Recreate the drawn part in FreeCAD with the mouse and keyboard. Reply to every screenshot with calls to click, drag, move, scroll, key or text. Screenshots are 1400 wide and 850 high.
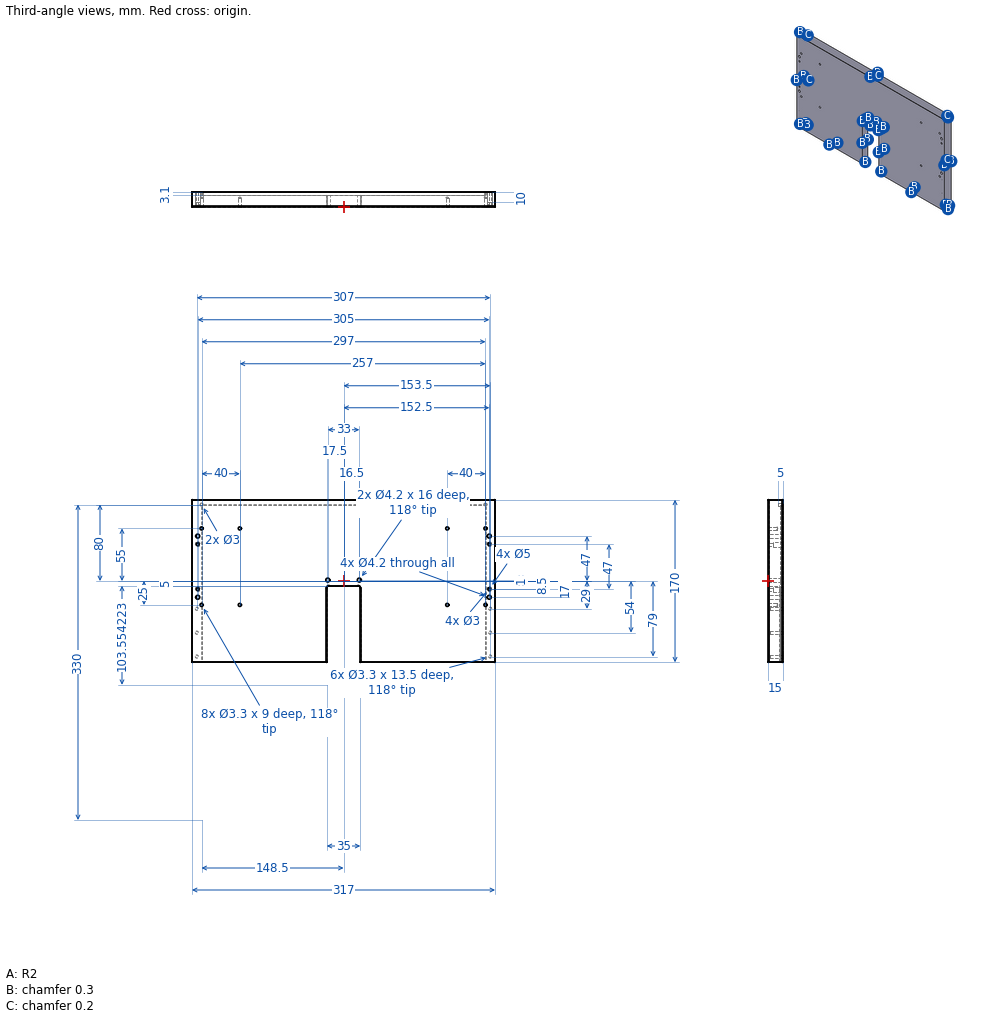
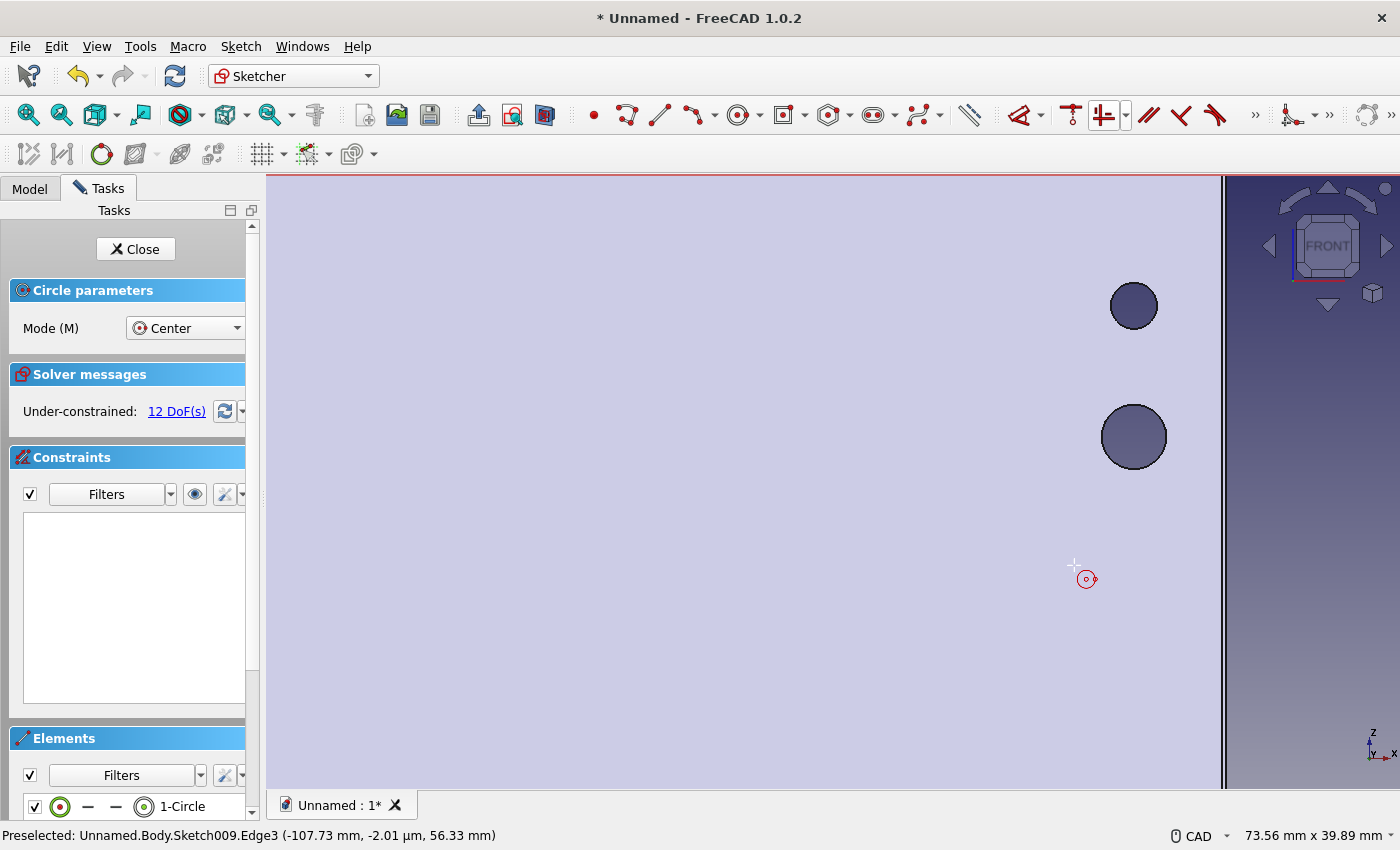
scroll(1075, 566, down, 10)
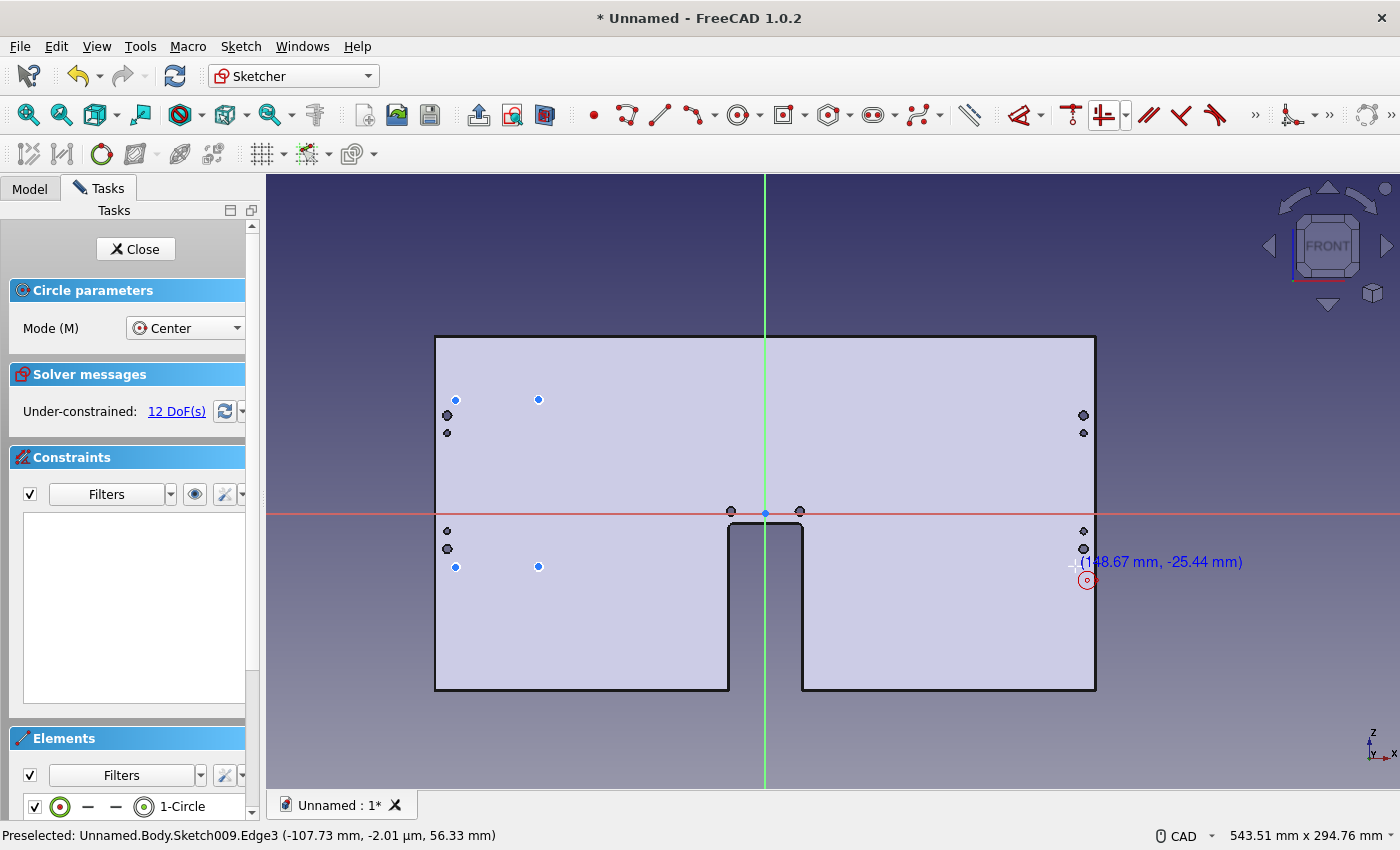
click(1075, 566)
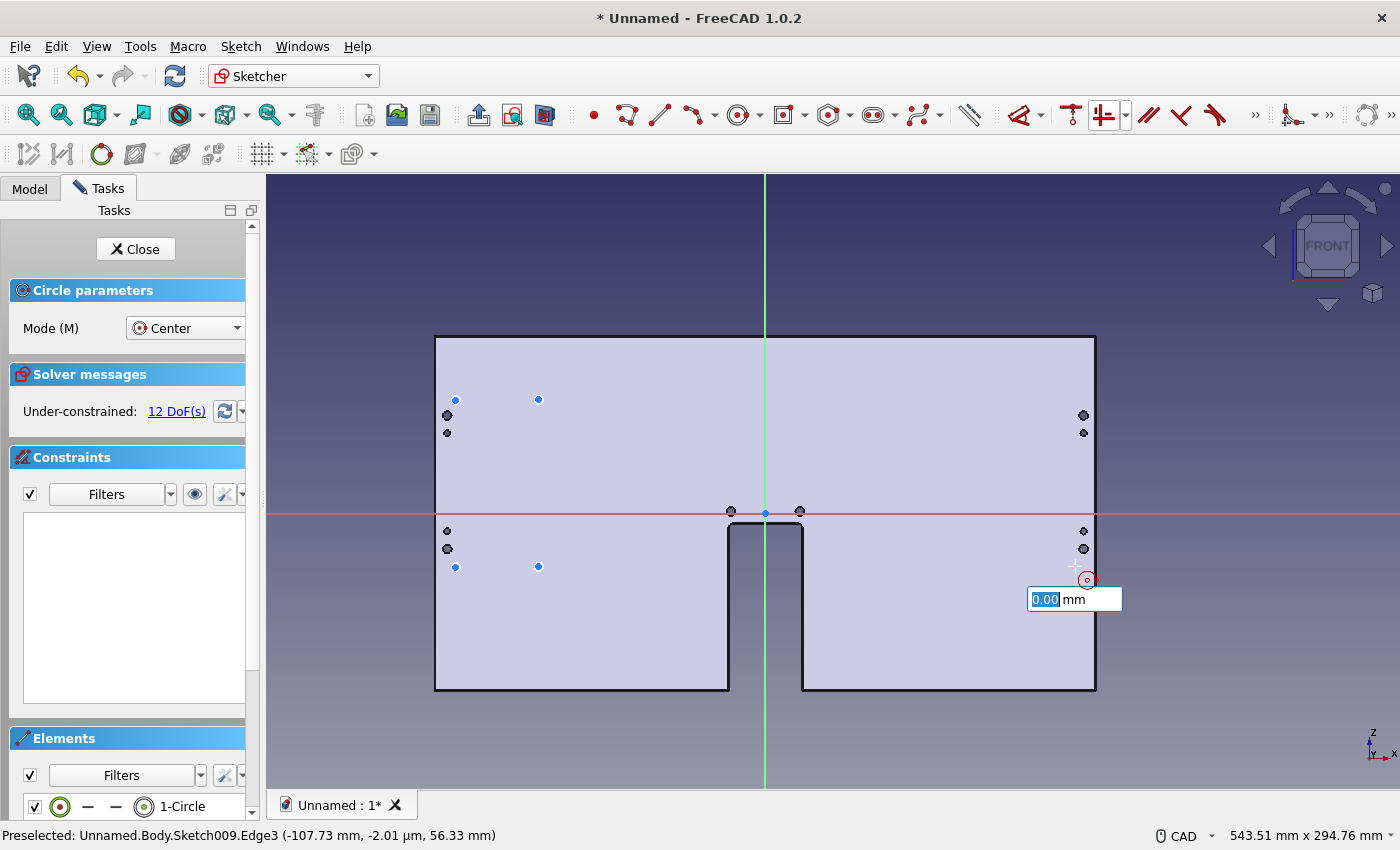
scroll(1078, 563, up, 8)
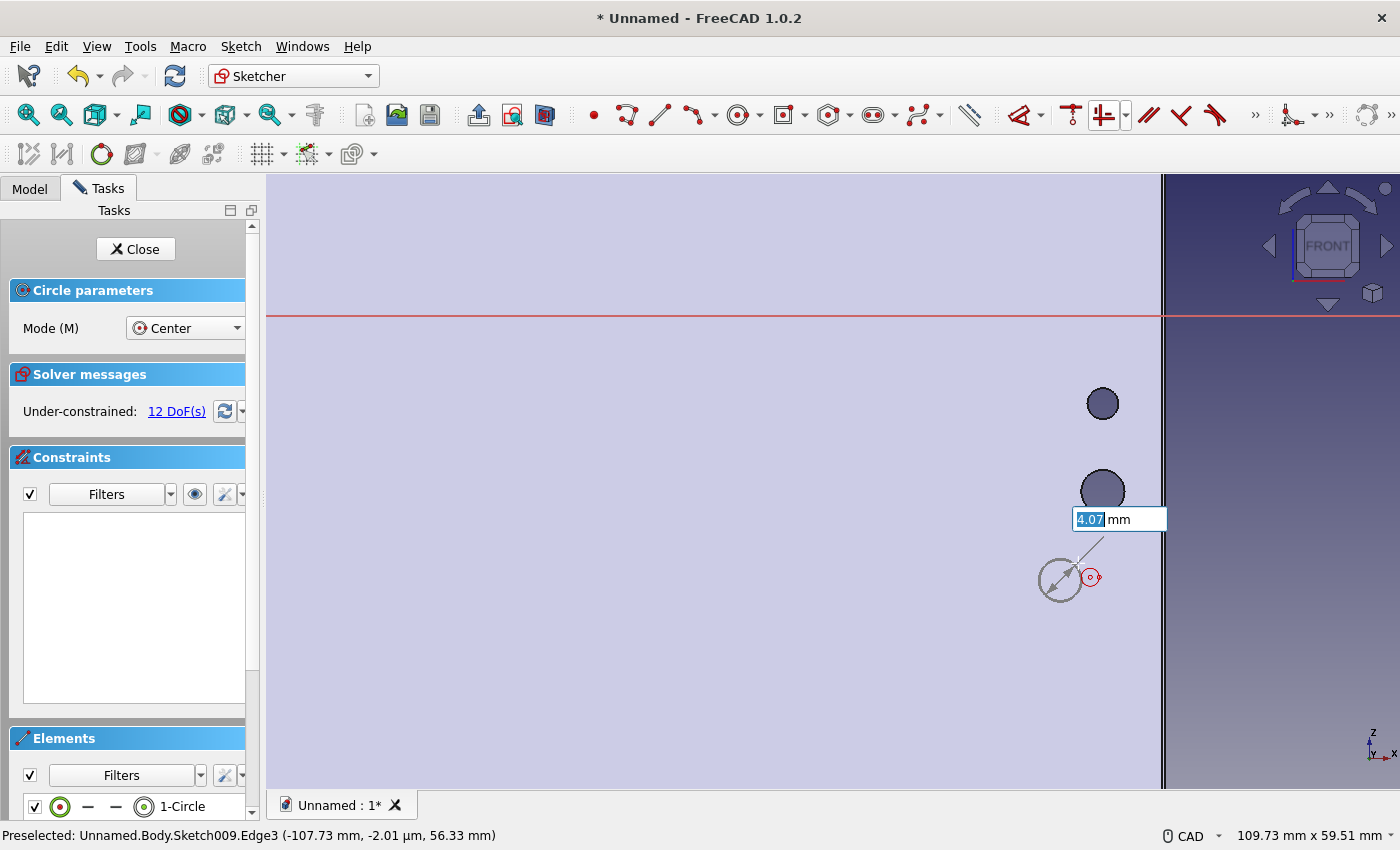
click(1074, 562)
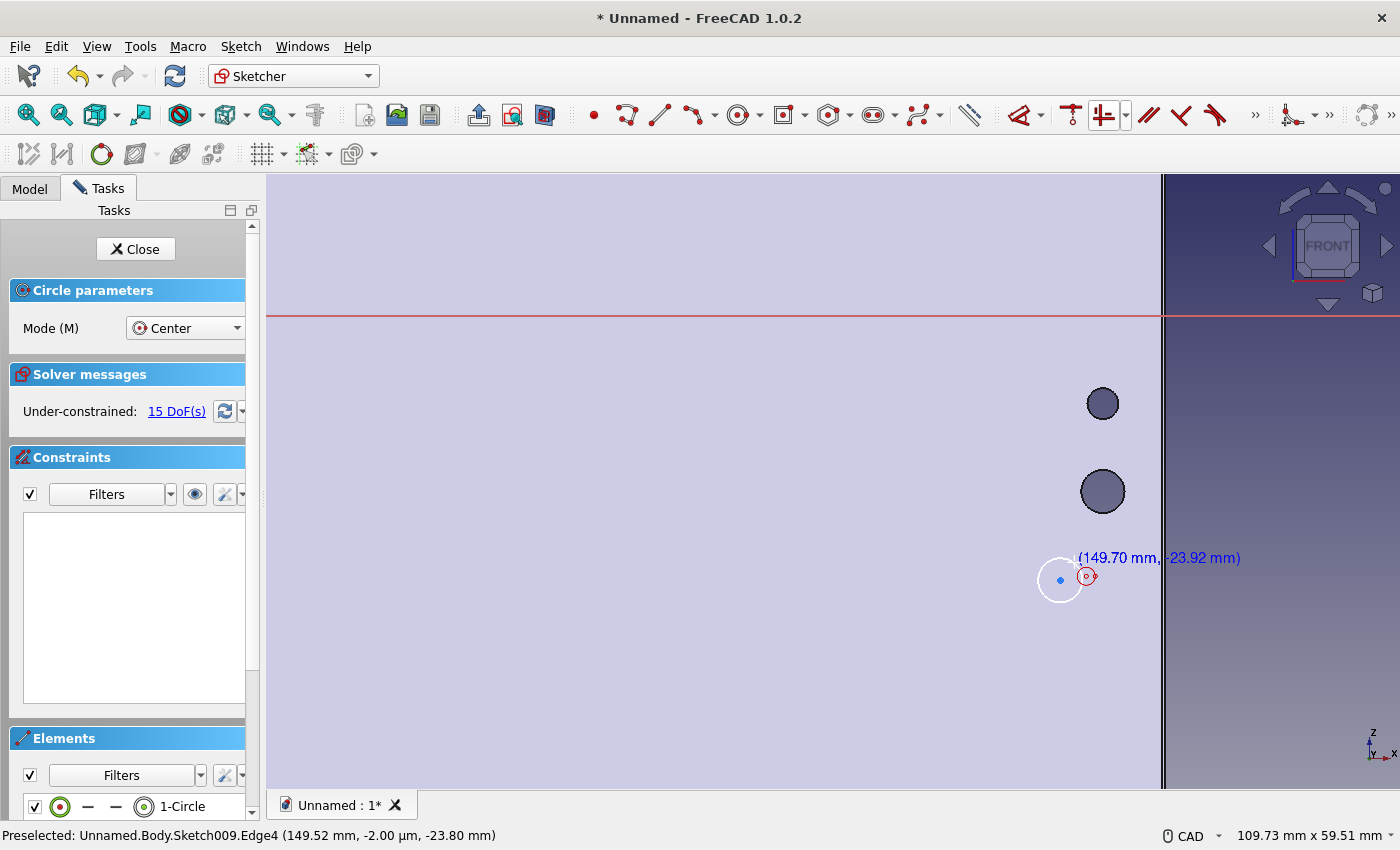
scroll(648, 574, up, 2)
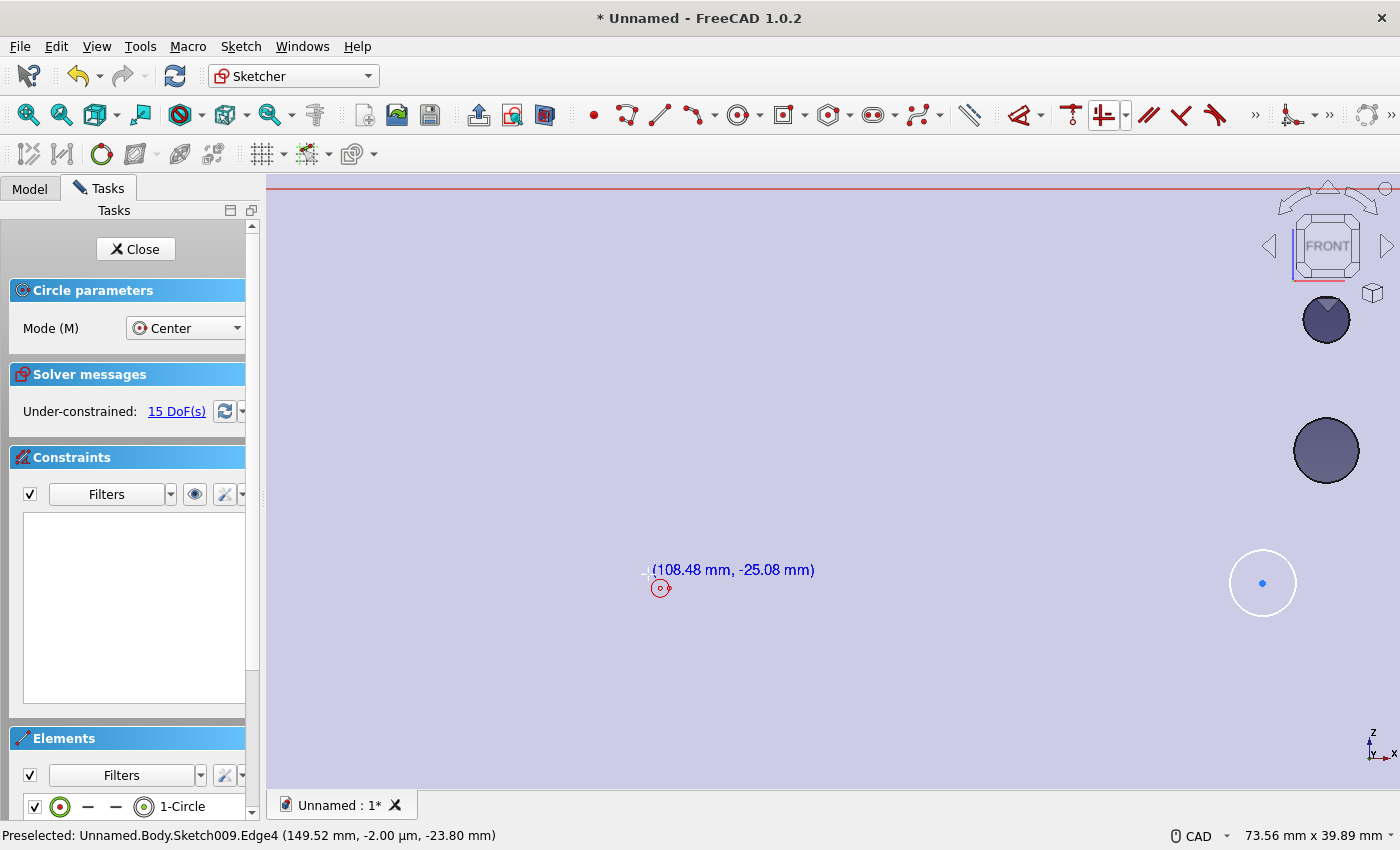
scroll(1045, 564, down, 10)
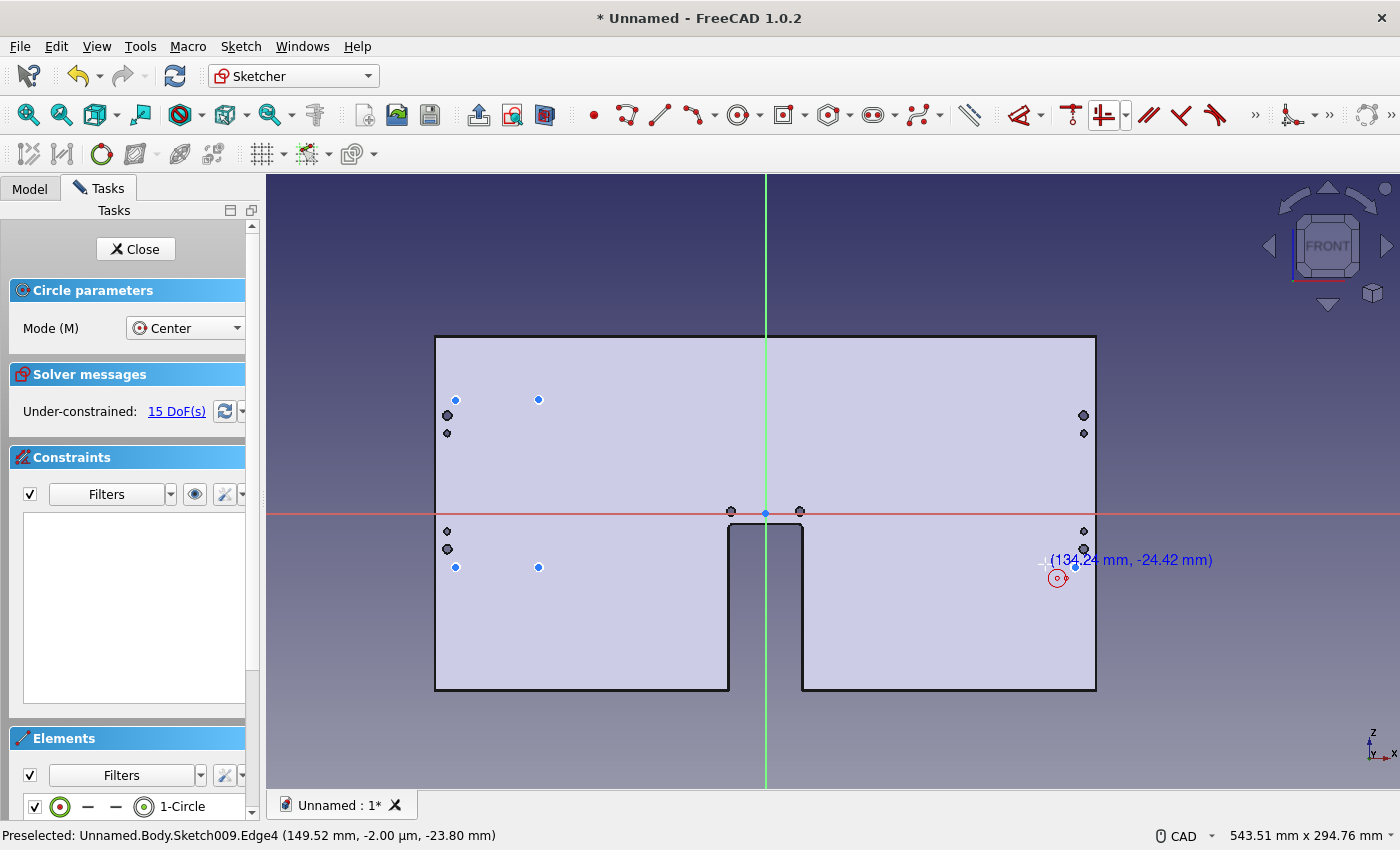
click(992, 566)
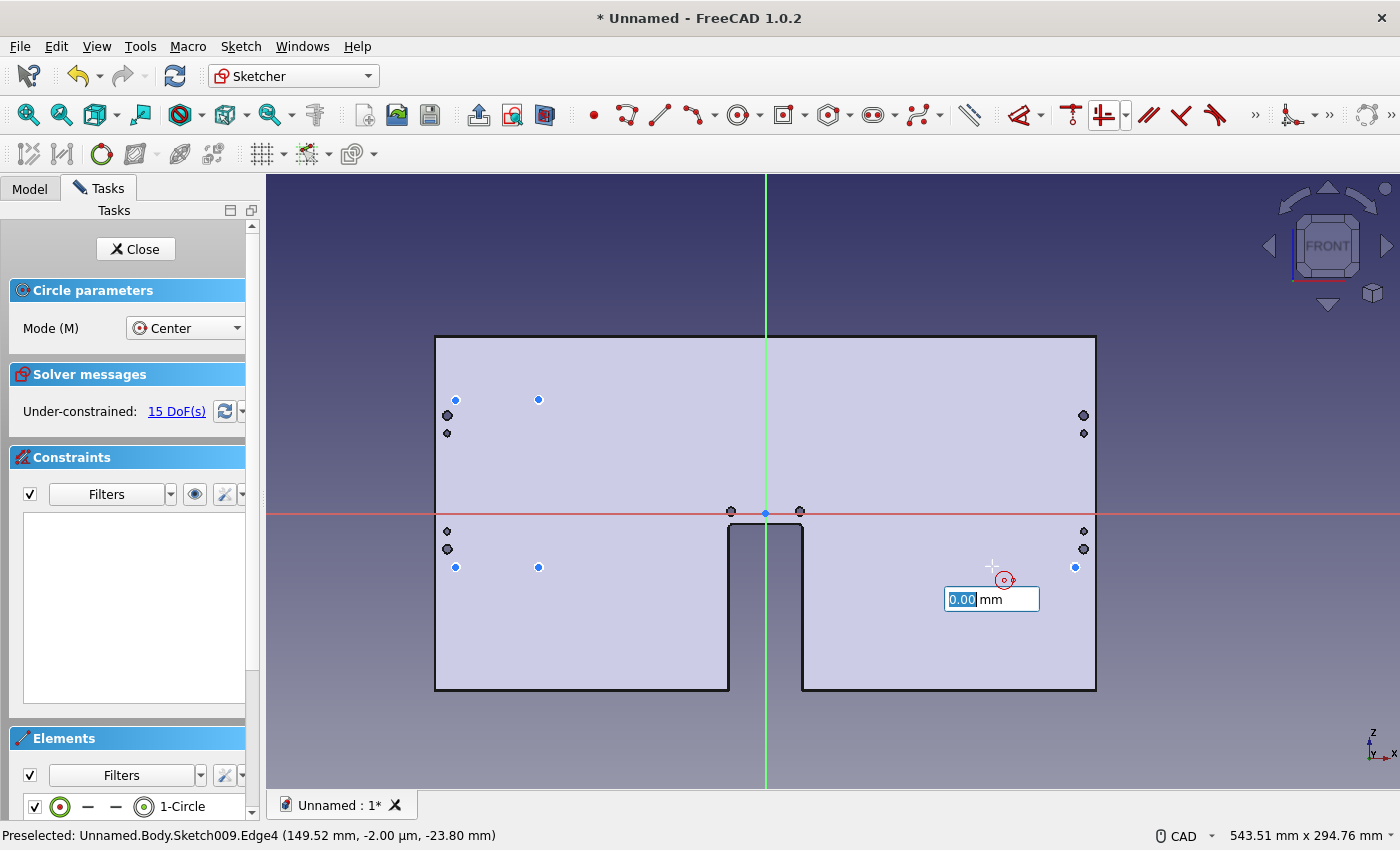
scroll(994, 563, up, 8)